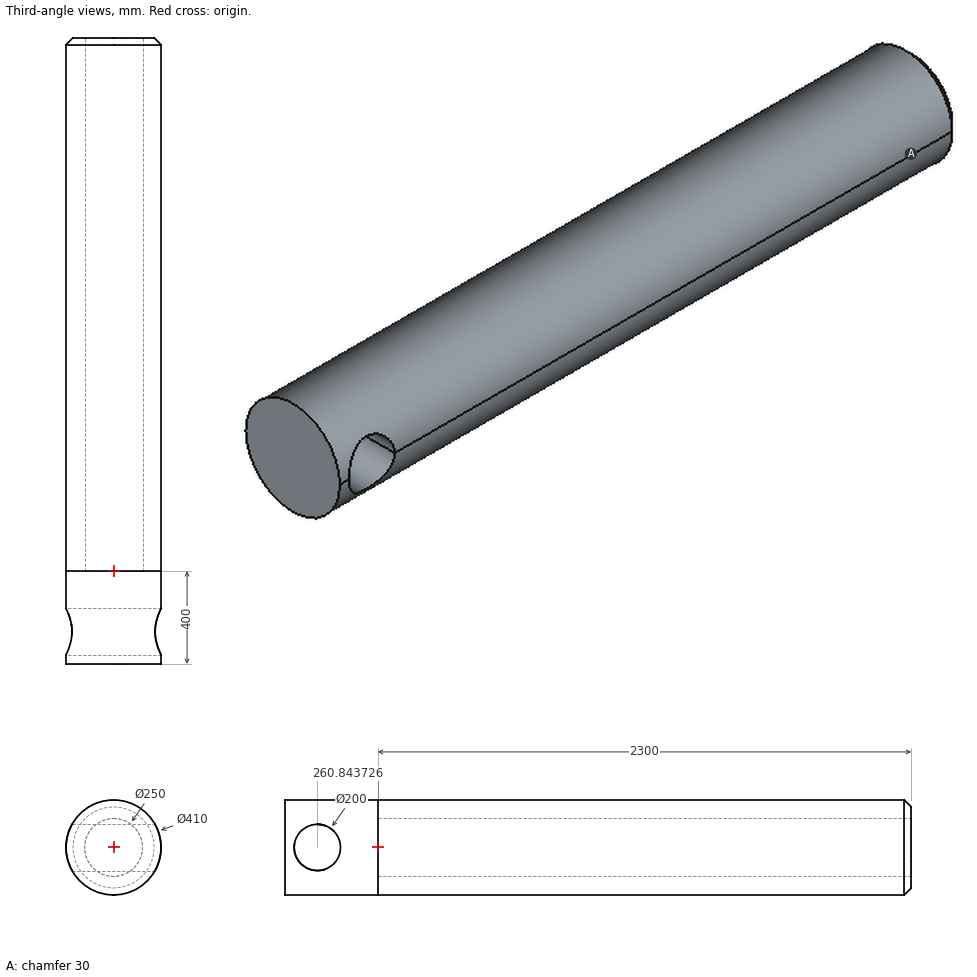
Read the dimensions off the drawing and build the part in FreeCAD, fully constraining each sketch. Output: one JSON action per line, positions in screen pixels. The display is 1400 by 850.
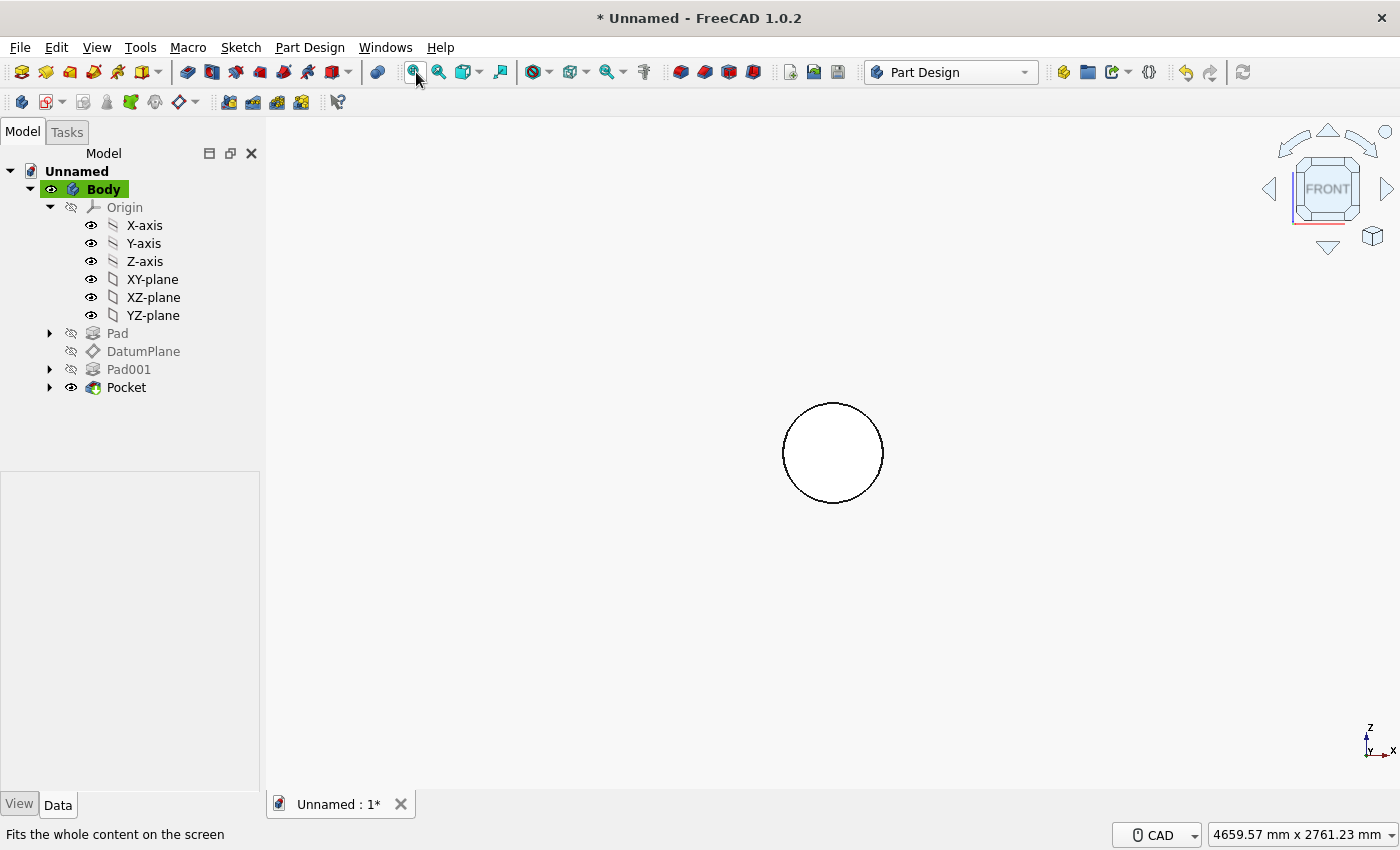
{"action": "key", "text": "3"}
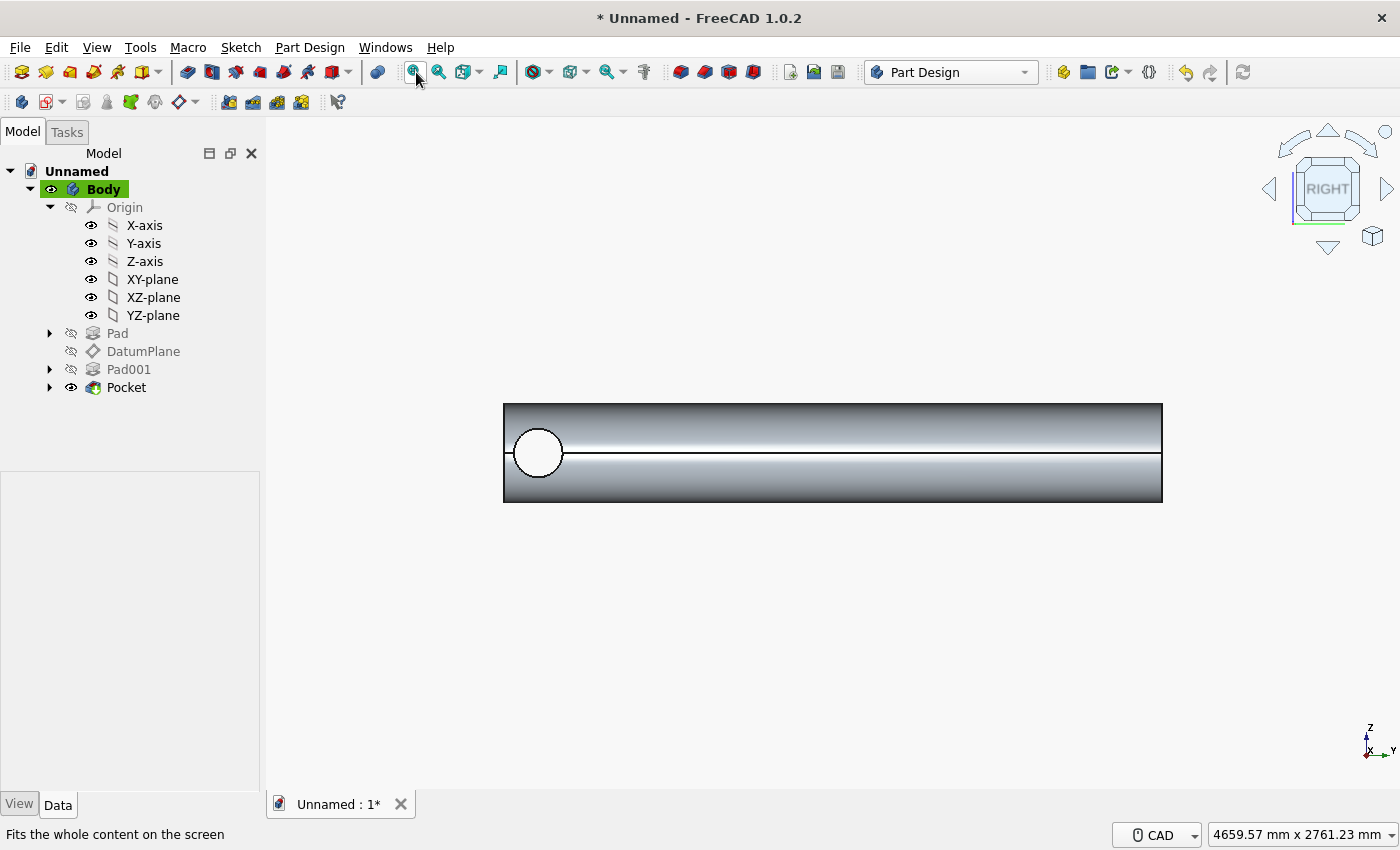
{"action": "left_click", "coordinate": [1162, 405]}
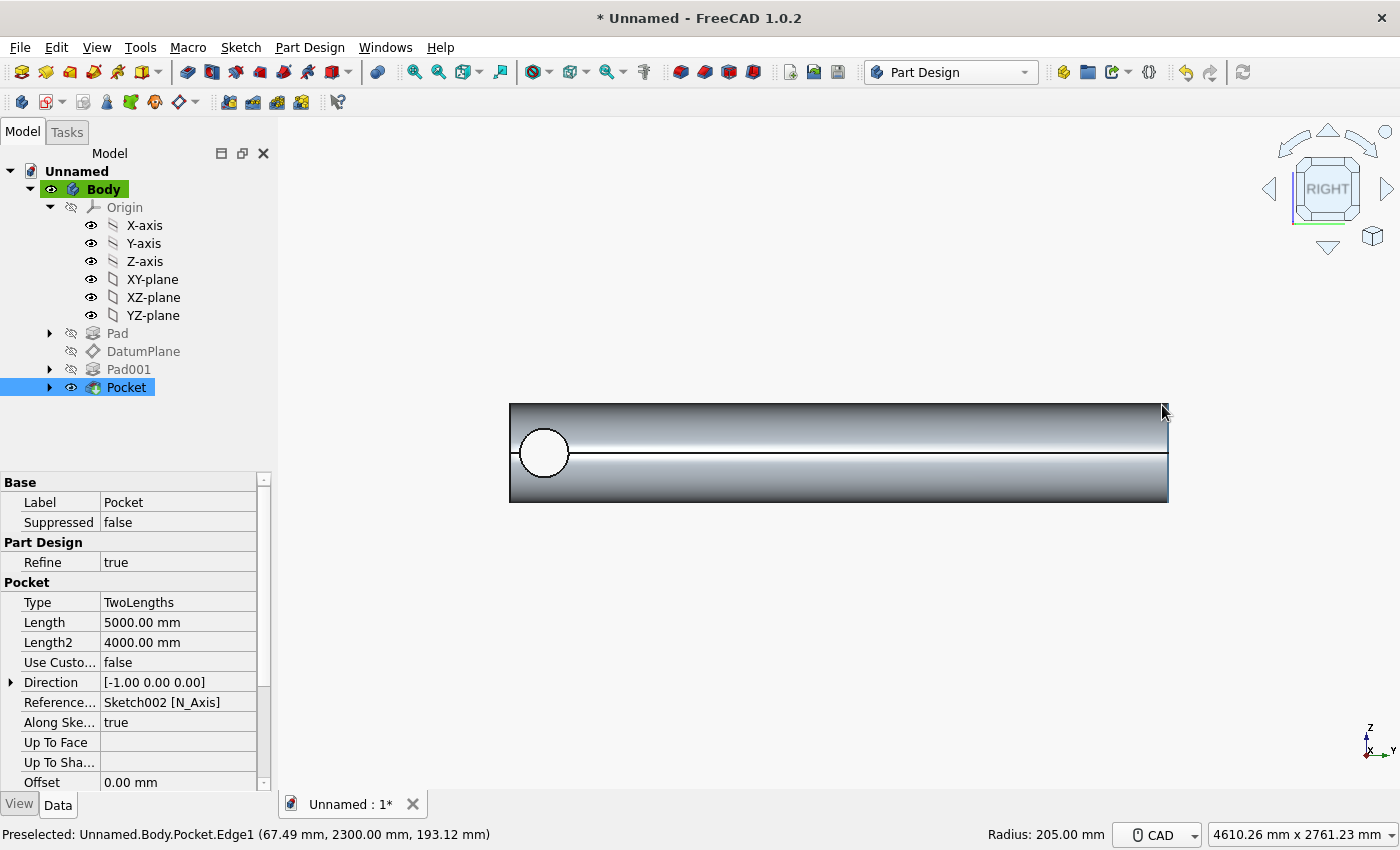
{"action": "left_click", "coordinate": [706, 72]}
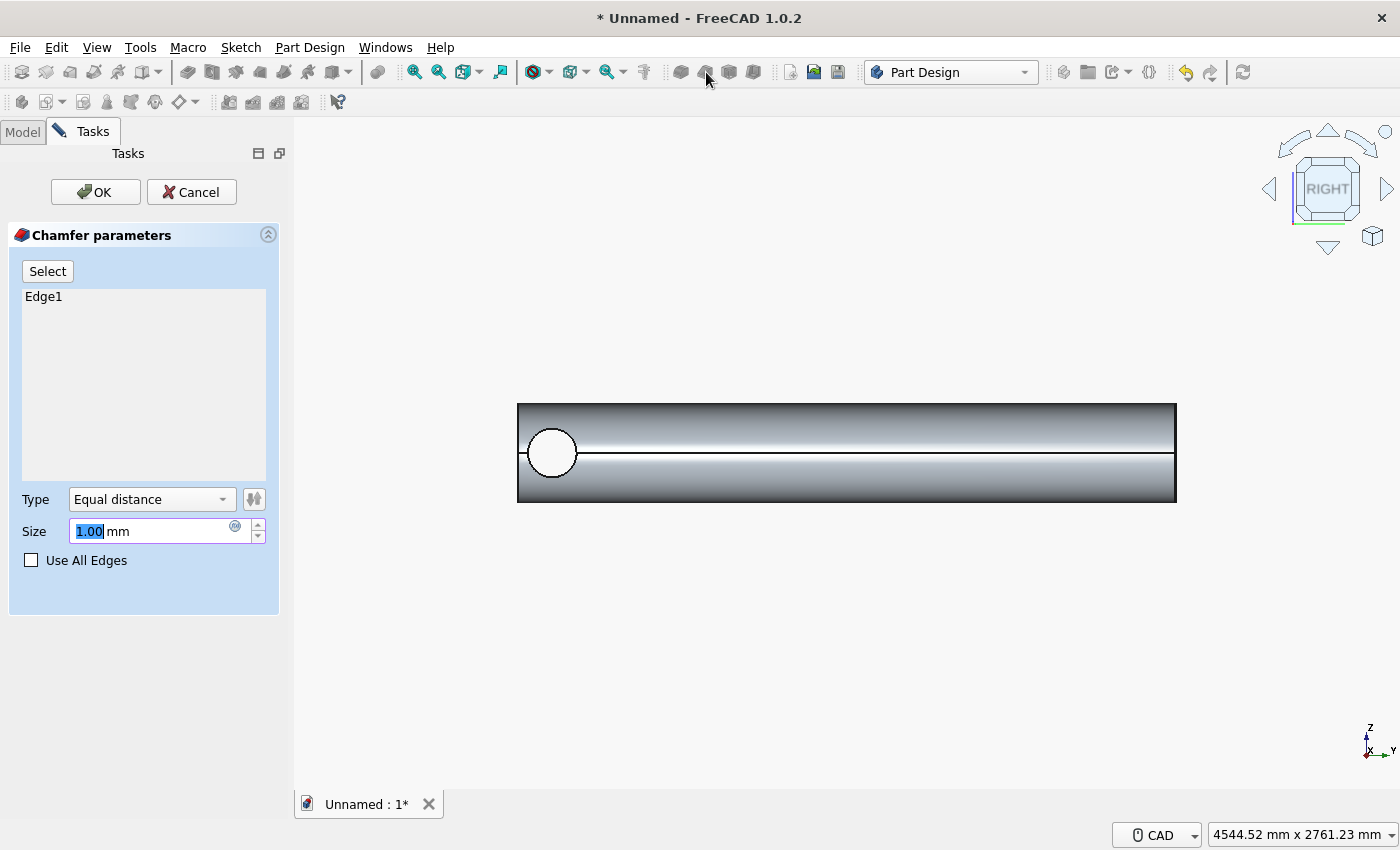
{"action": "type", "text": "30"}
{"action": "key", "text": "Tab"}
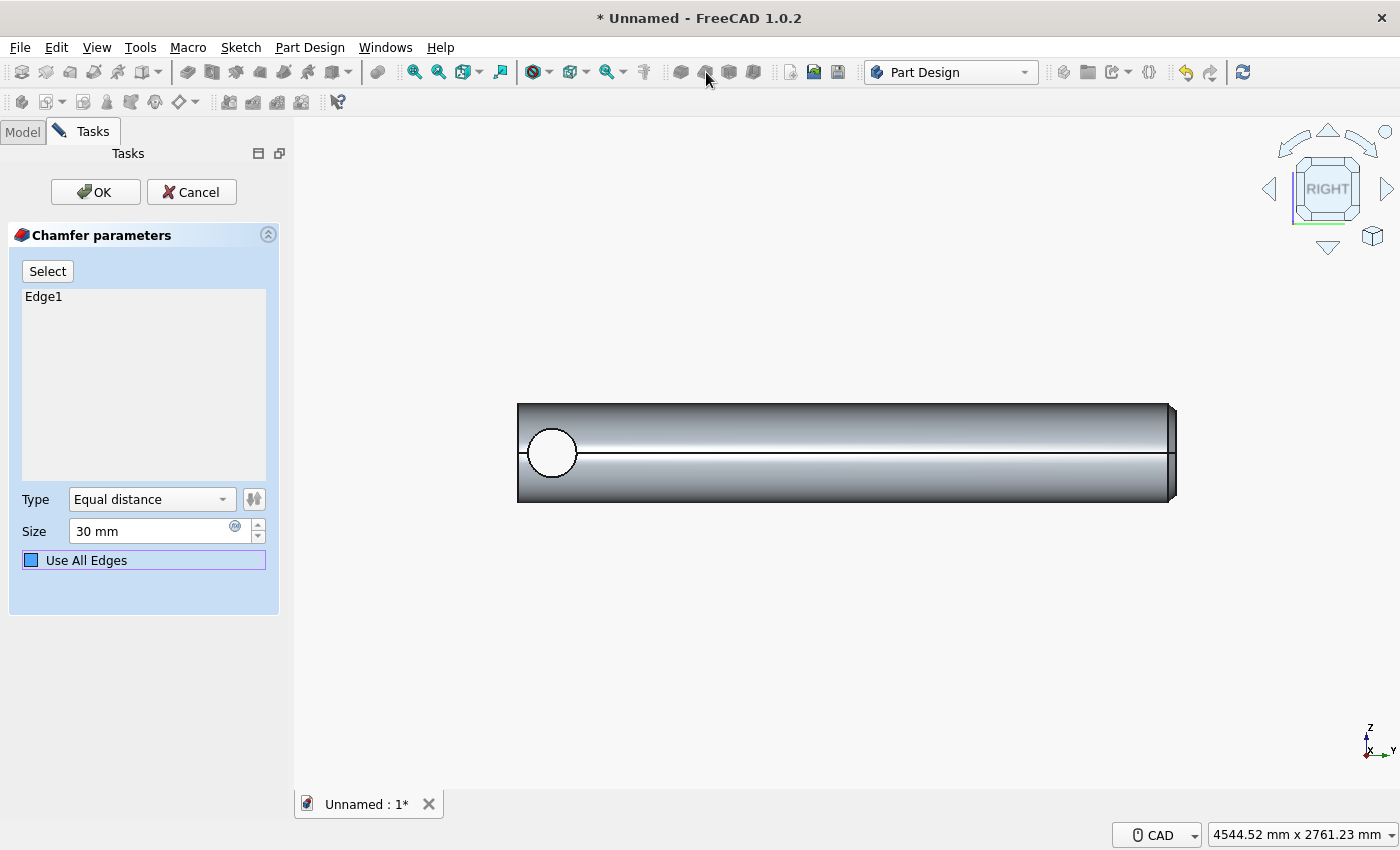
{"action": "left_click", "coordinate": [96, 192]}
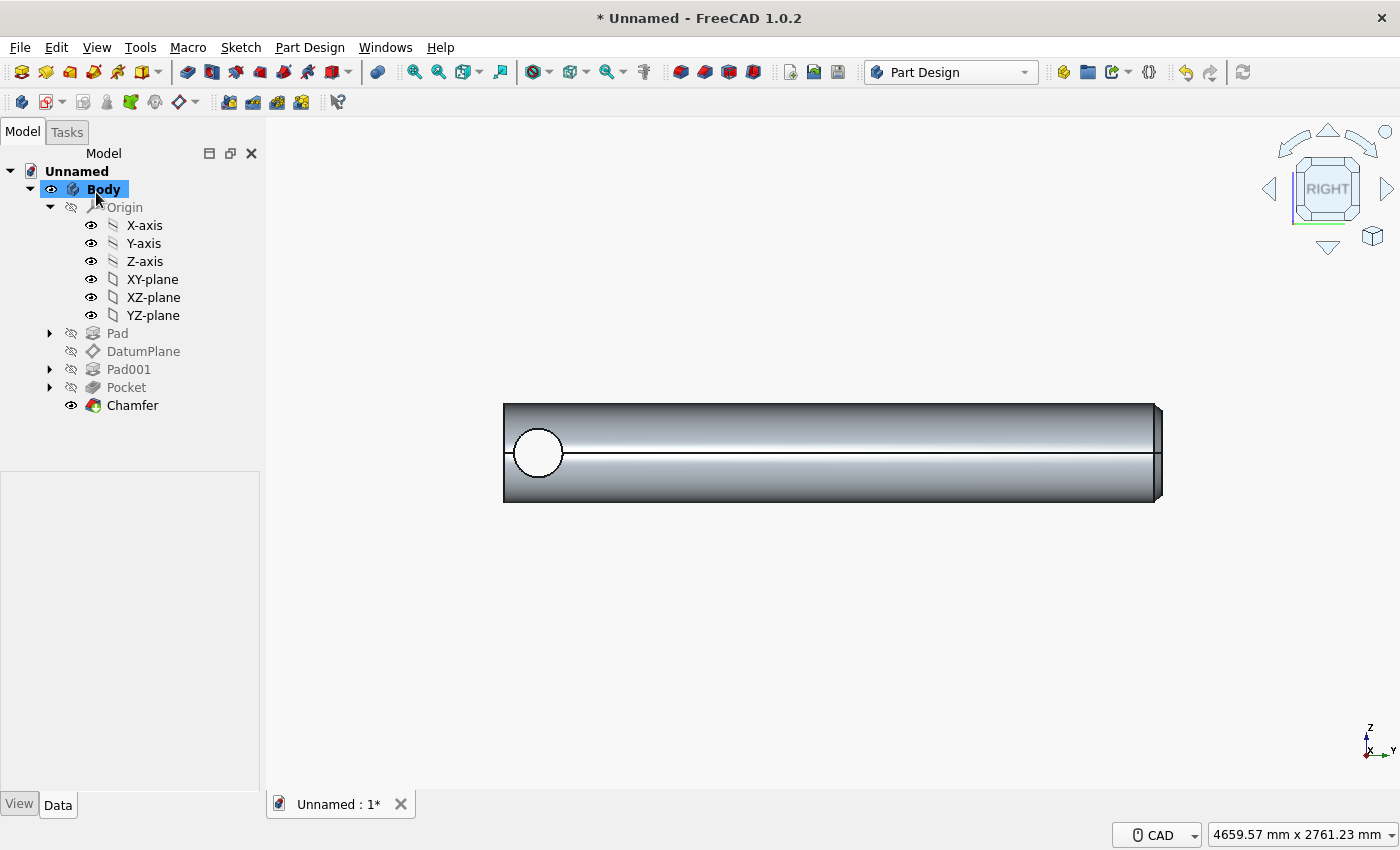
{"action": "key", "text": "0"}